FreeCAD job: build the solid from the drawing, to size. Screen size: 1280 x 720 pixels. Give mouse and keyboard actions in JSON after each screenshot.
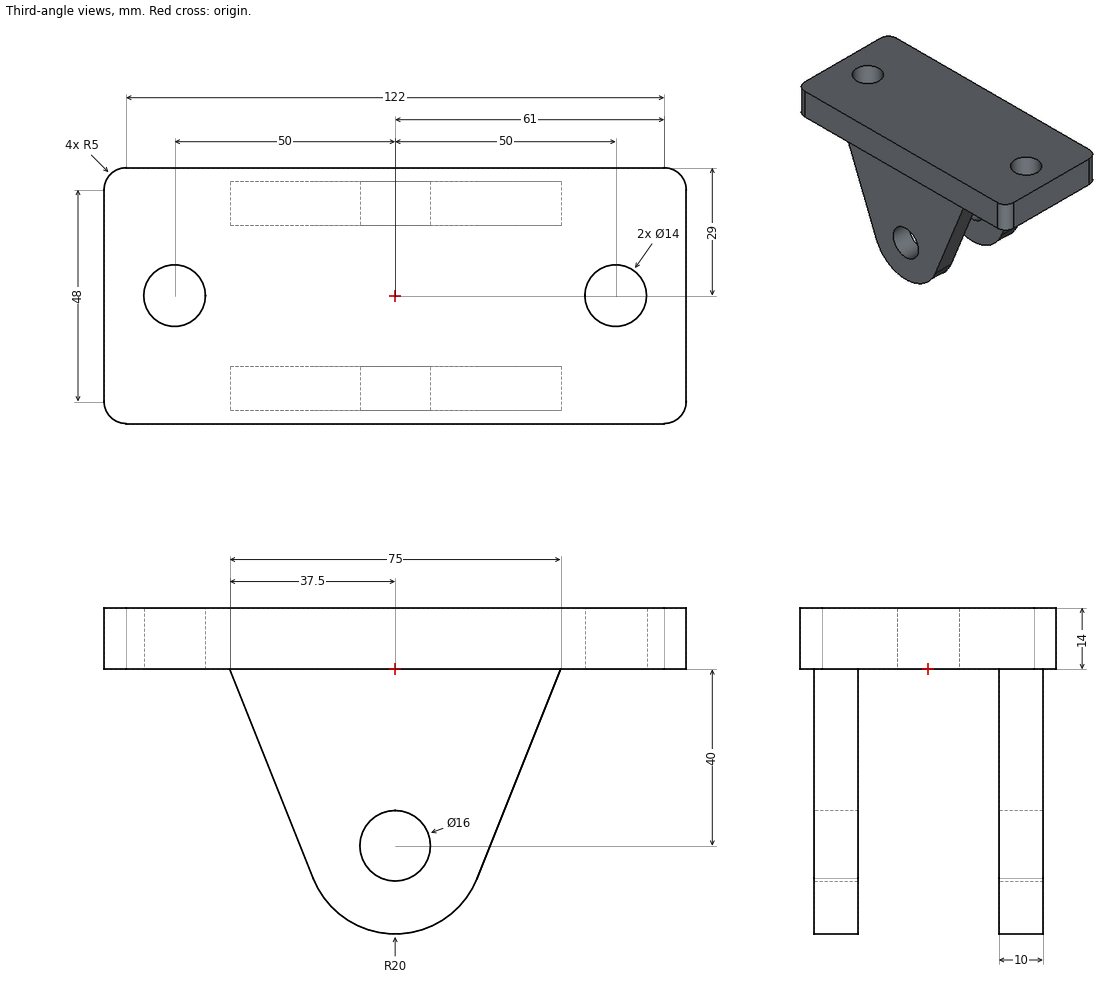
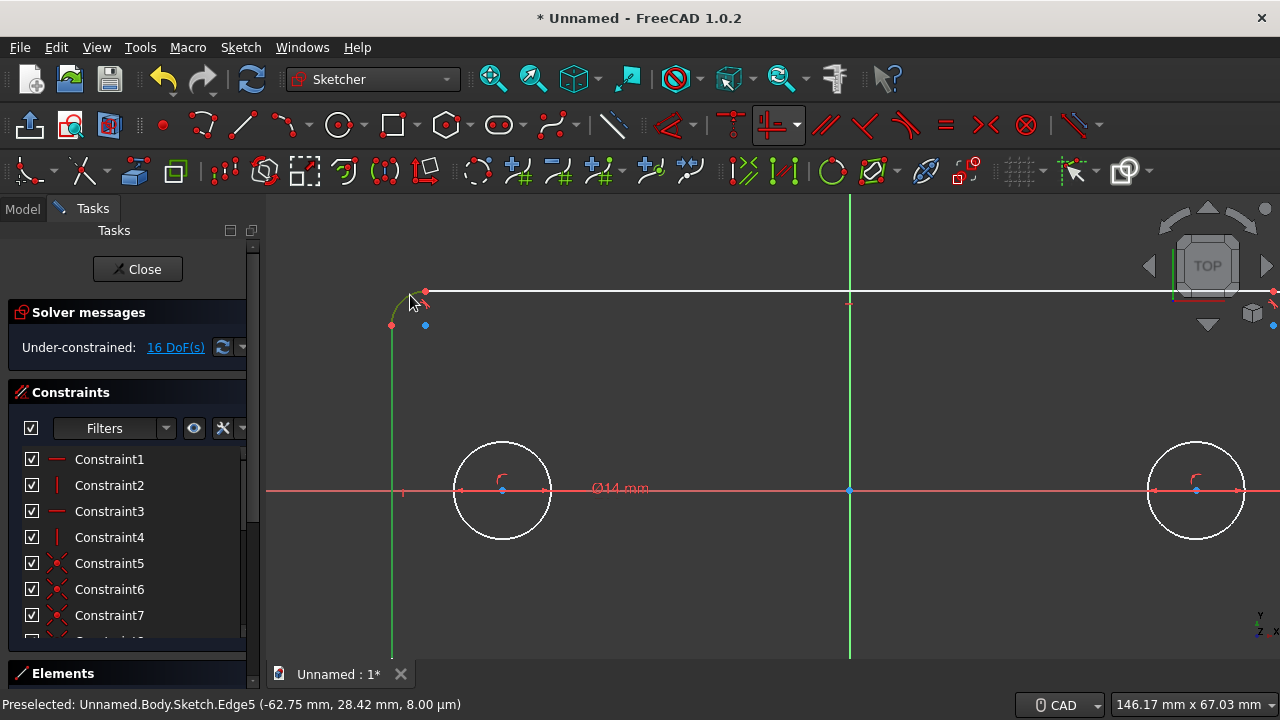
{"action": "left_click", "coordinate": [906, 126]}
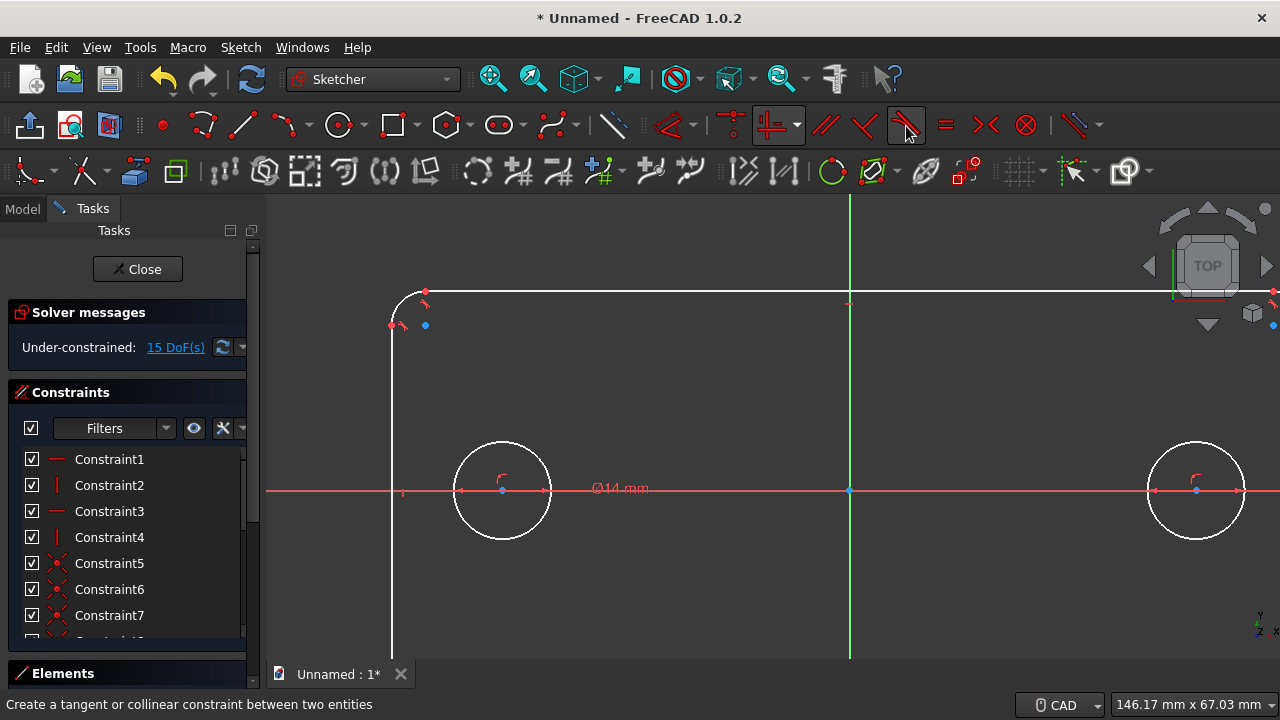
{"action": "left_click", "coordinate": [392, 426]}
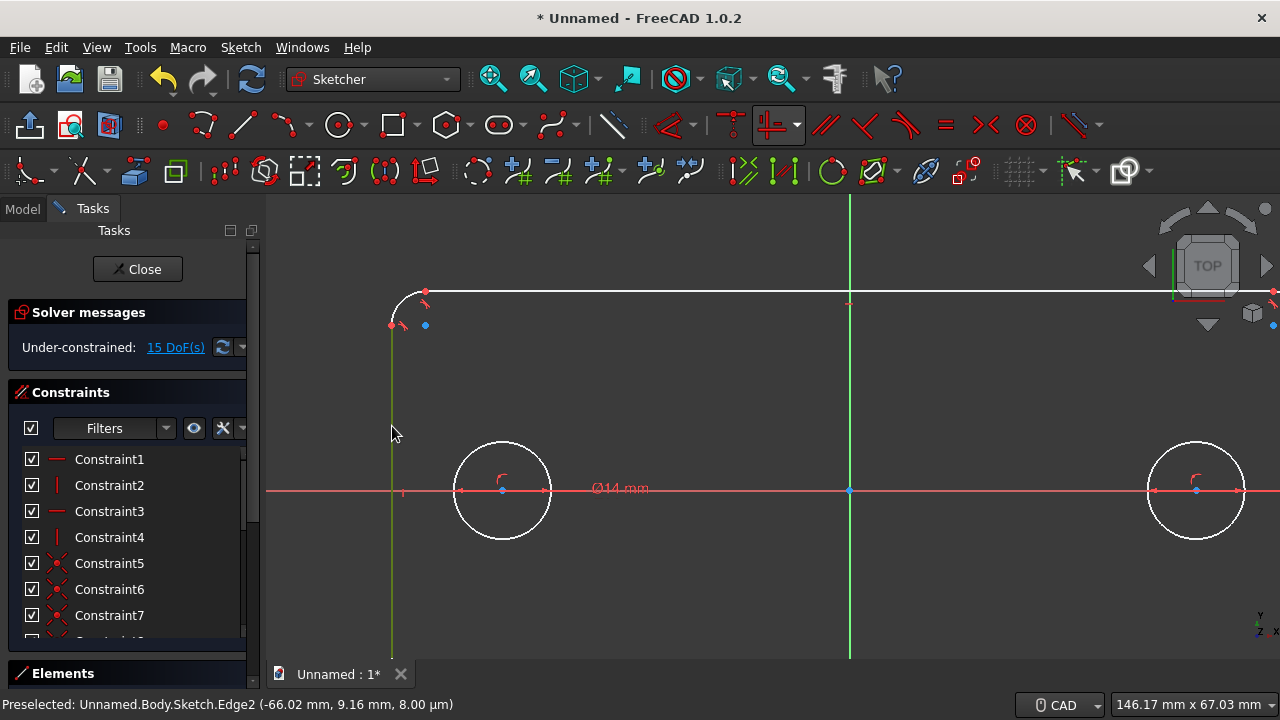
{"action": "scroll", "coordinate": [410, 296], "scroll_direction": "down", "scroll_amount": 2}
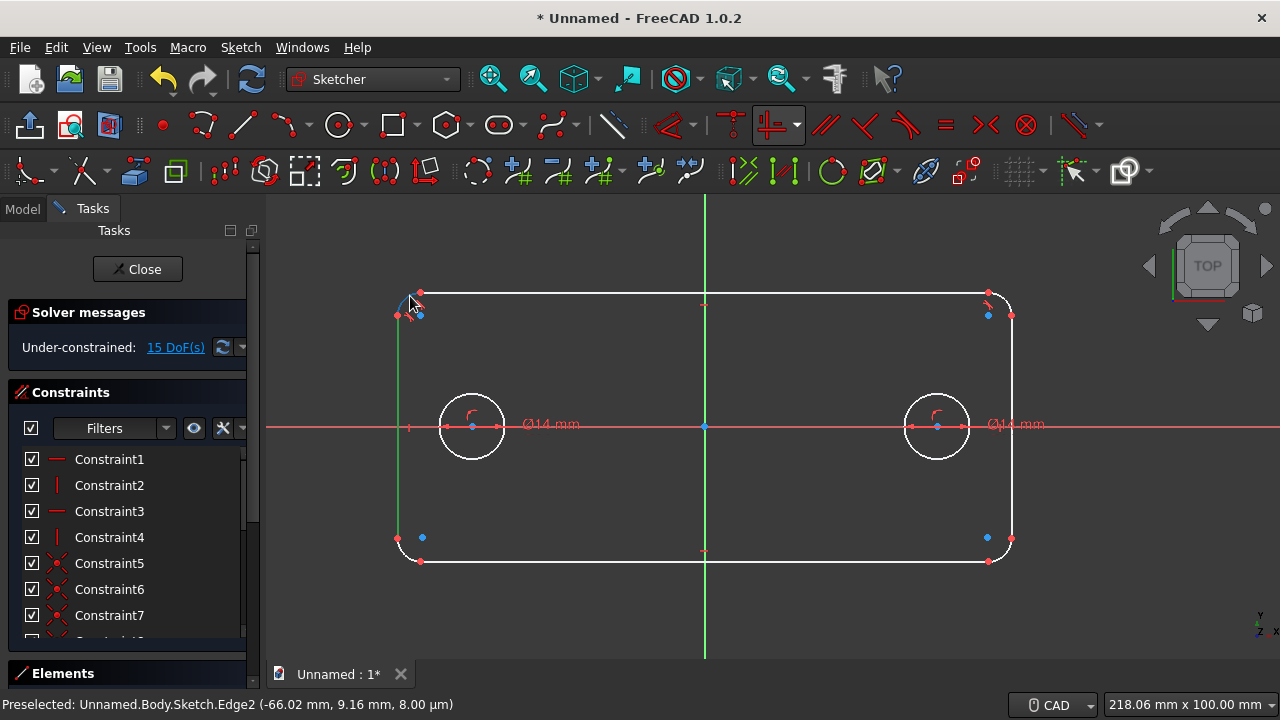
{"action": "scroll", "coordinate": [401, 549], "scroll_direction": "up", "scroll_amount": 2}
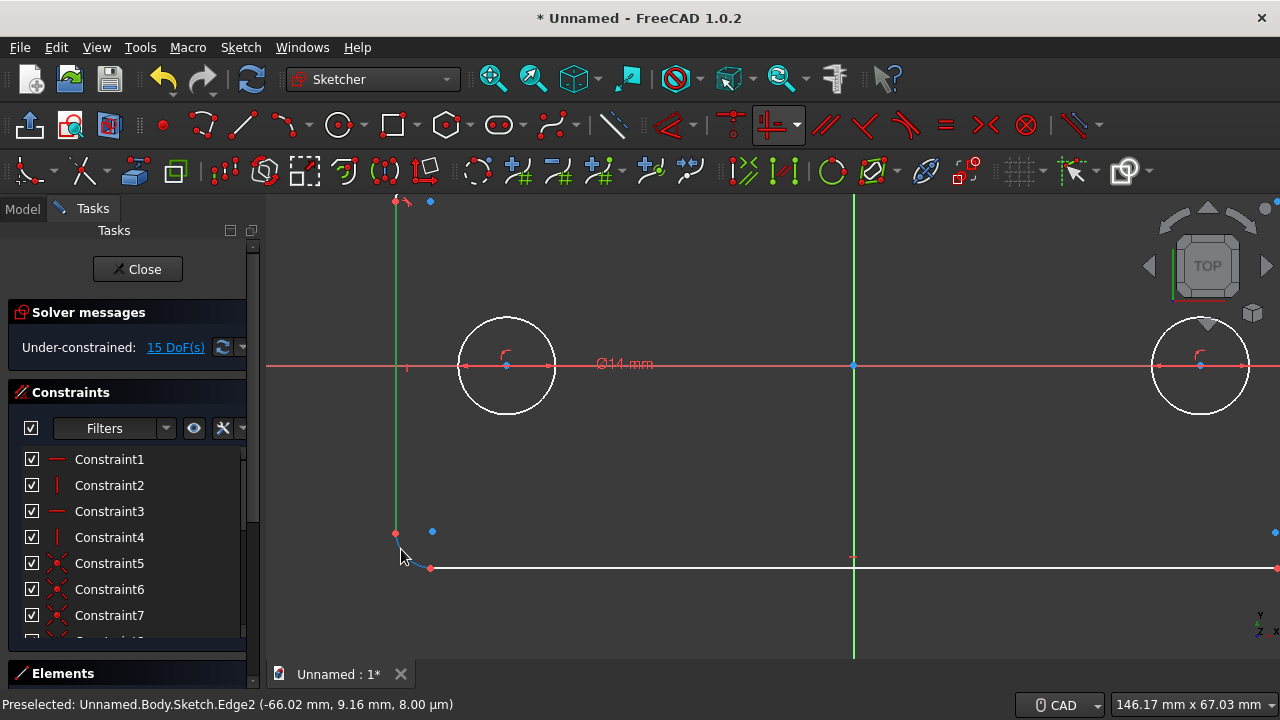
{"action": "left_click", "coordinate": [400, 549]}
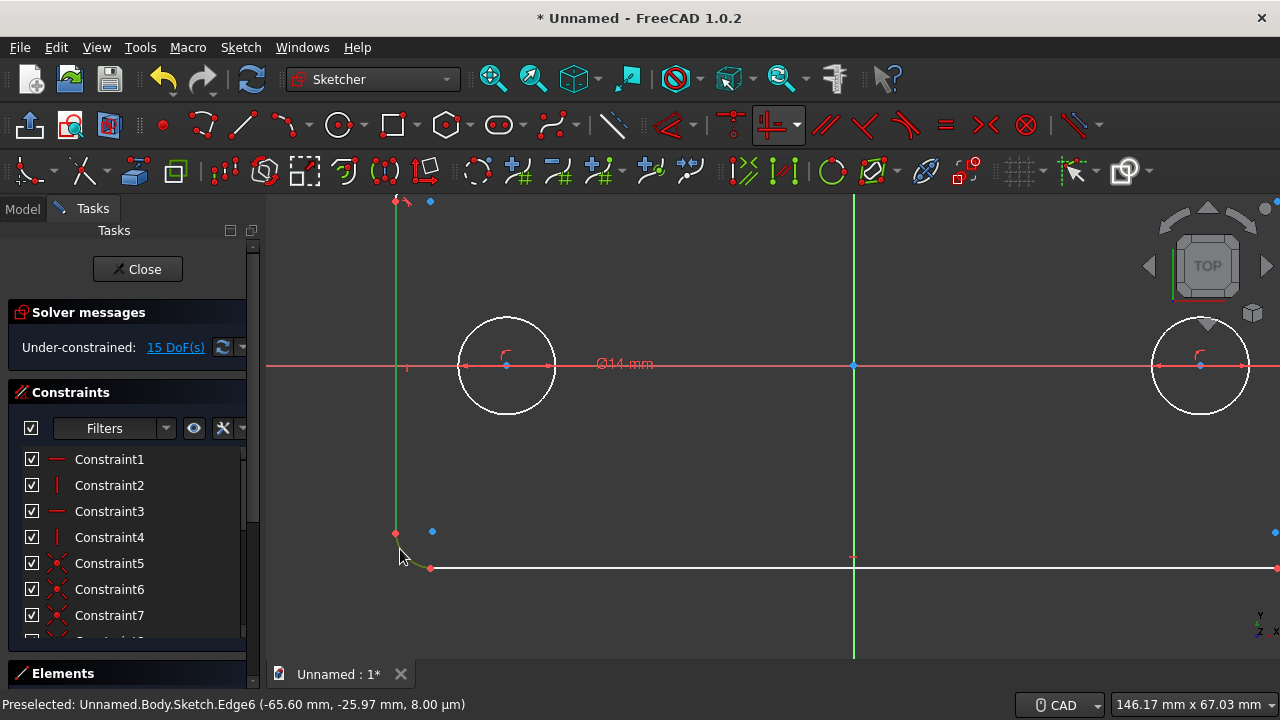
{"action": "left_click", "coordinate": [906, 126]}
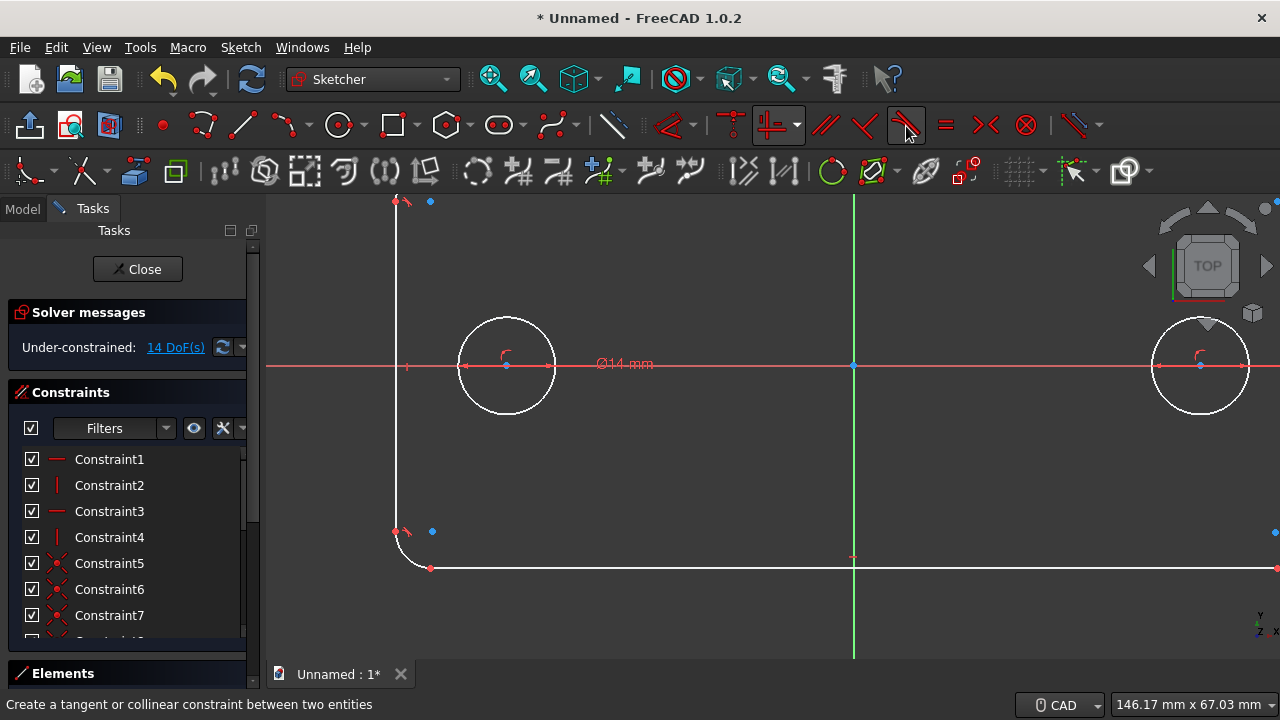
{"action": "left_click", "coordinate": [684, 568]}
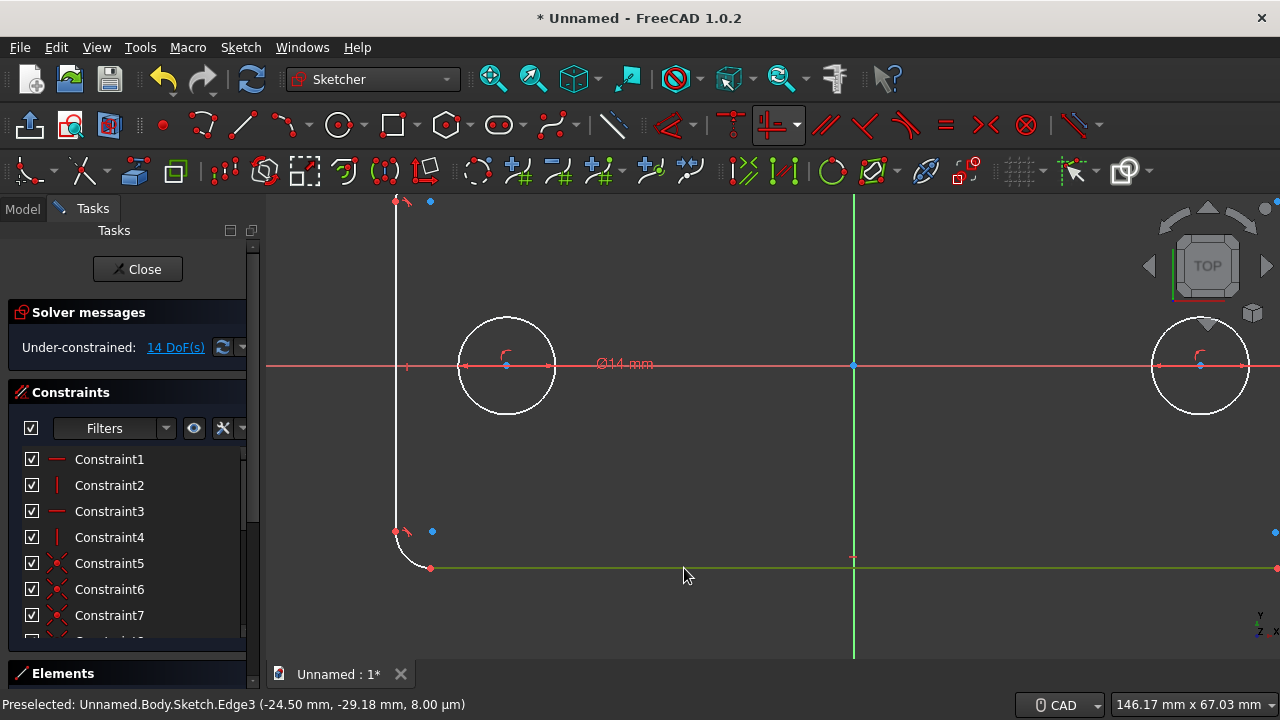
{"action": "left_click", "coordinate": [400, 548]}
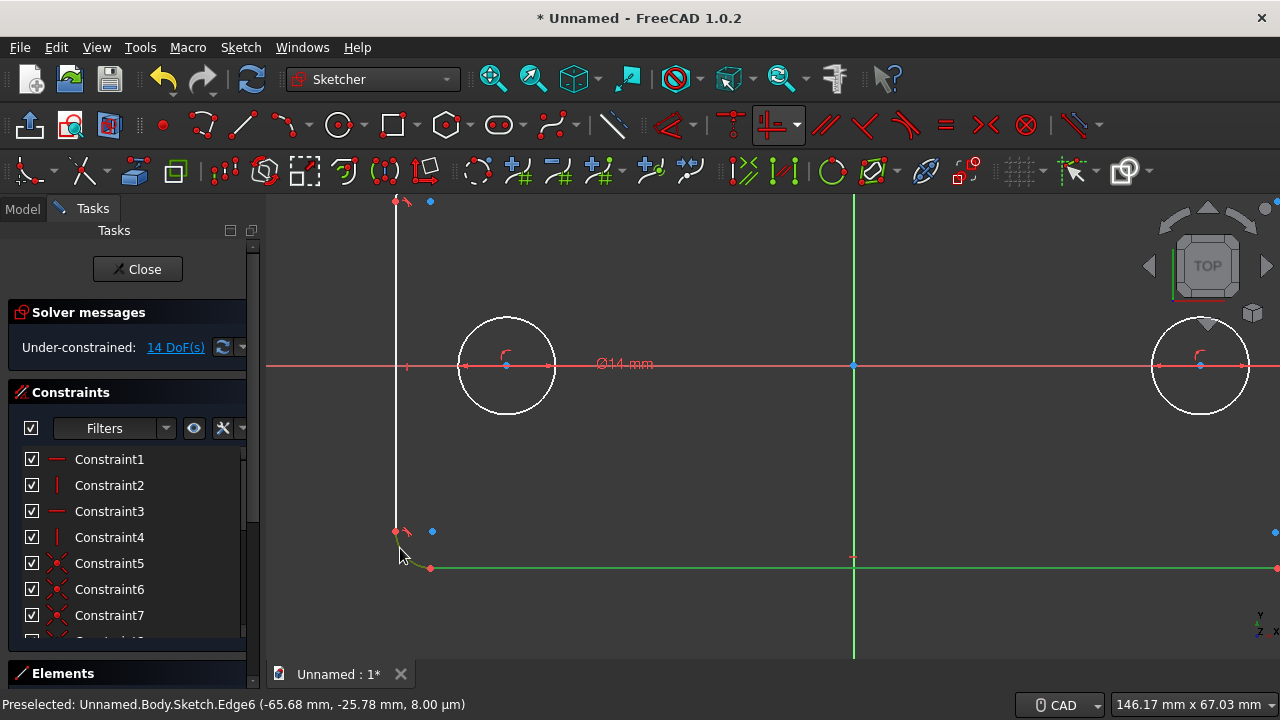
{"action": "left_click", "coordinate": [906, 126]}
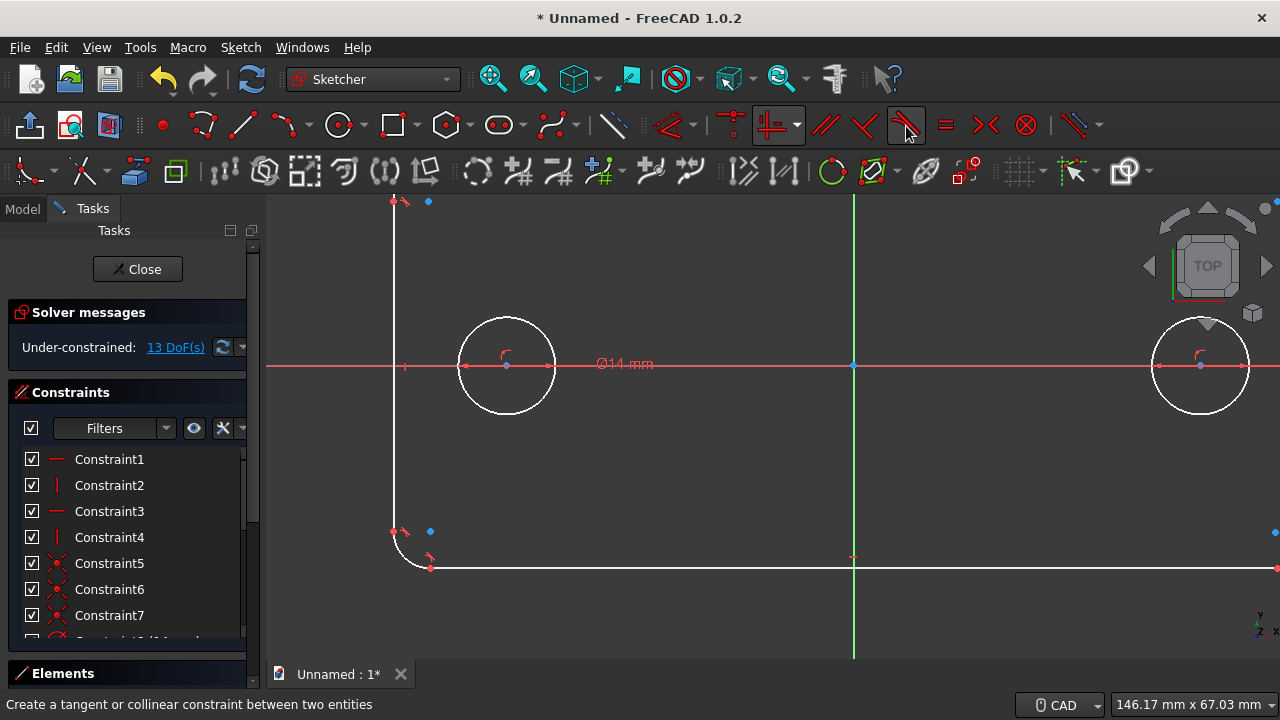
{"action": "left_click", "coordinate": [684, 568]}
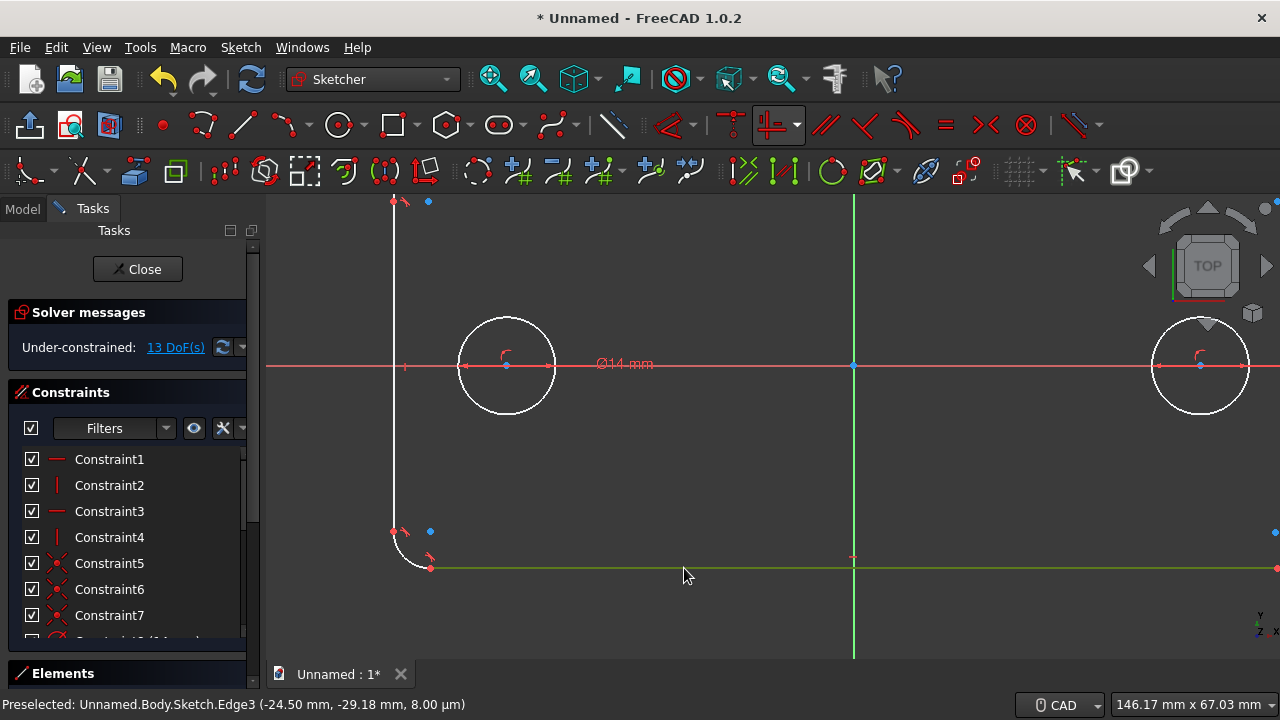
{"action": "scroll", "coordinate": [401, 550], "scroll_direction": "down", "scroll_amount": 2}